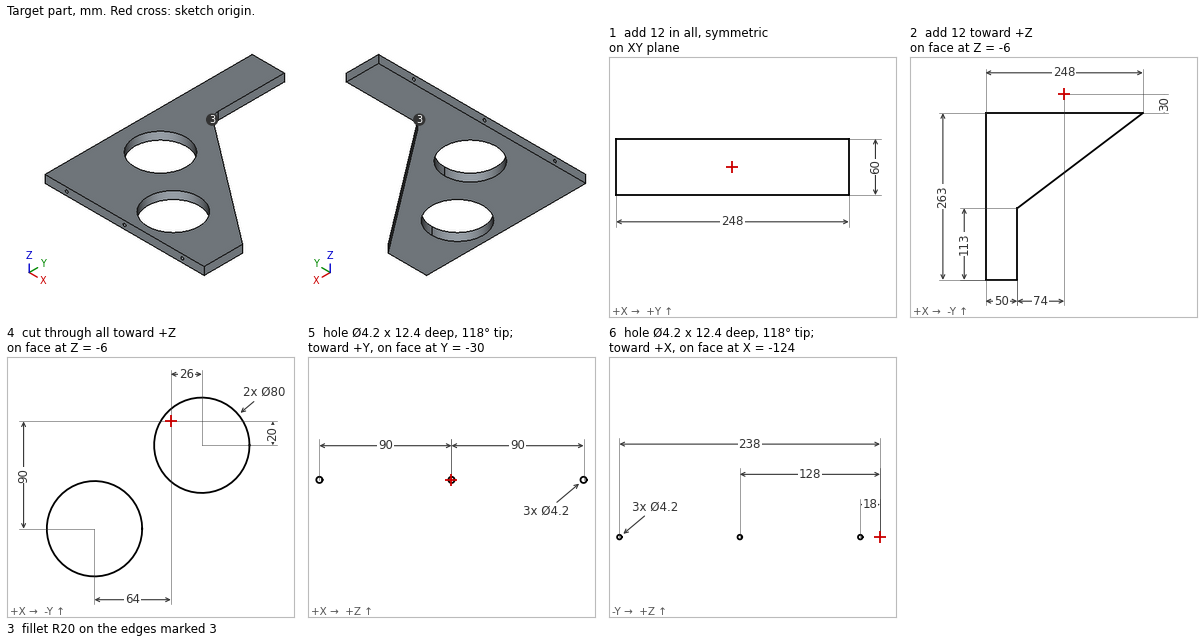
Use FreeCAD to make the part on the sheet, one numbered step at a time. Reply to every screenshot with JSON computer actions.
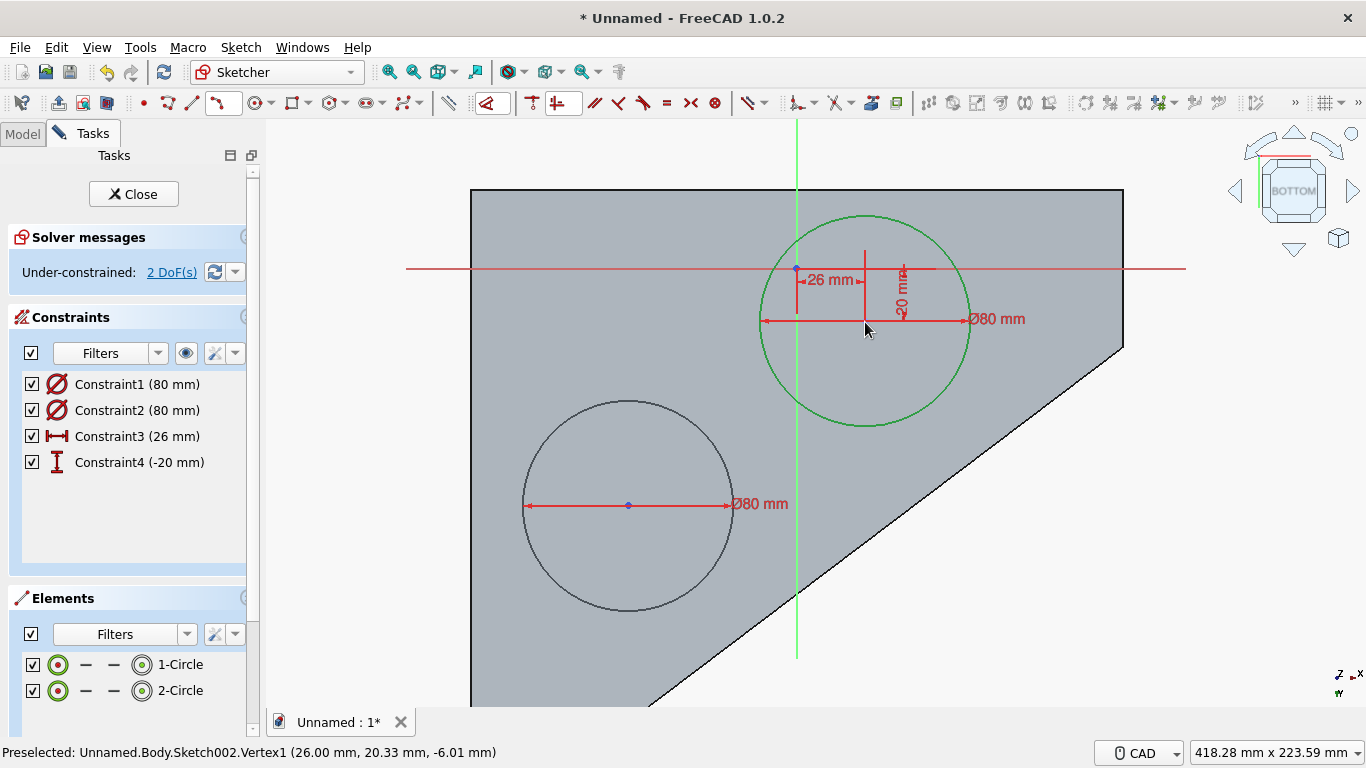
{"action": "left_click", "coordinate": [628, 506]}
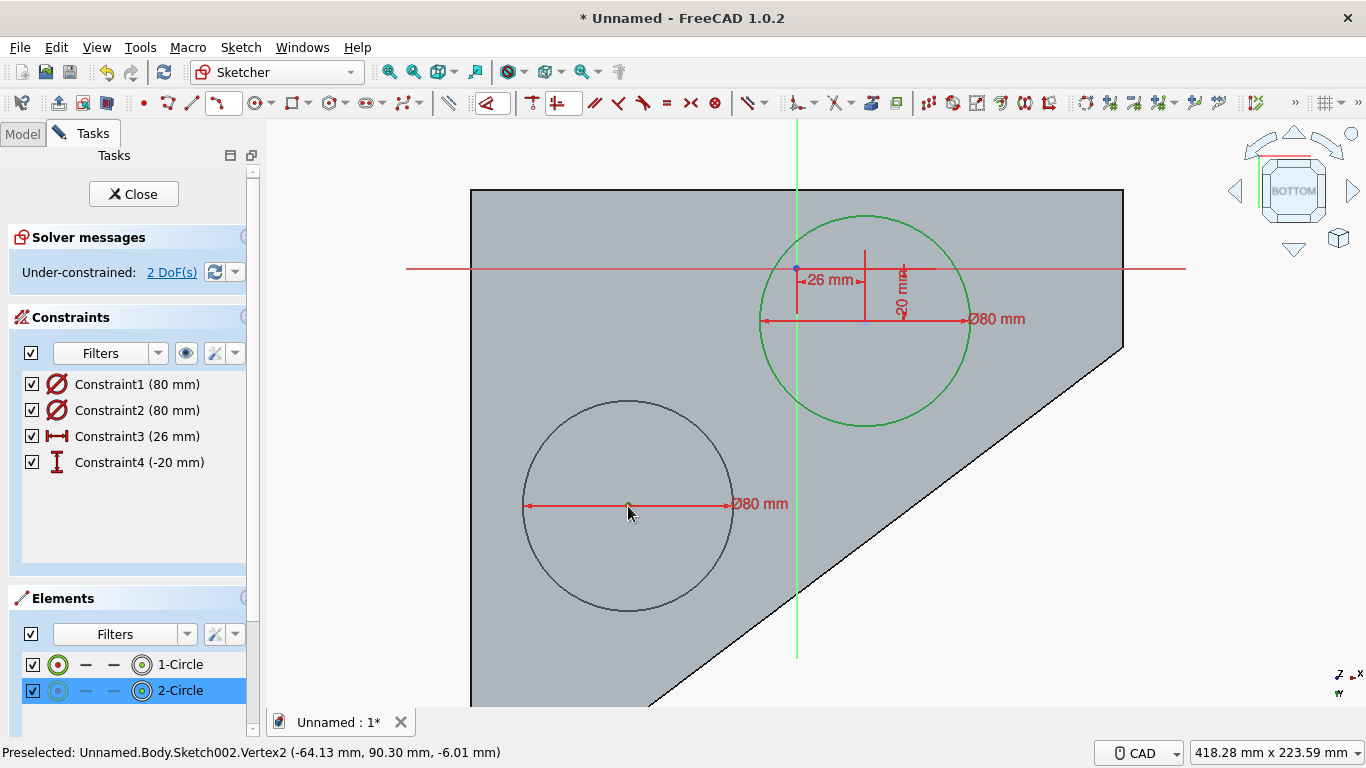
{"action": "key", "text": "l"}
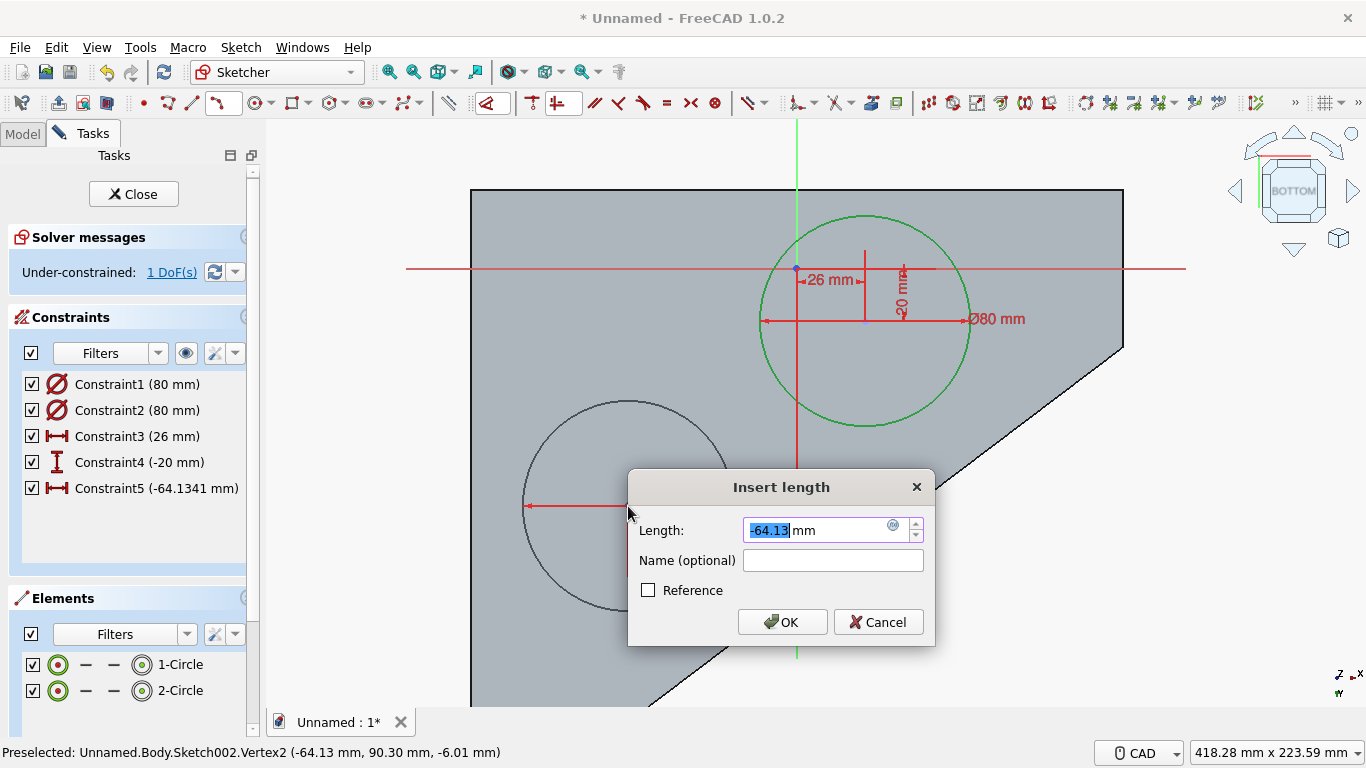
{"action": "type", "text": "-64"}
{"action": "key", "text": "Return"}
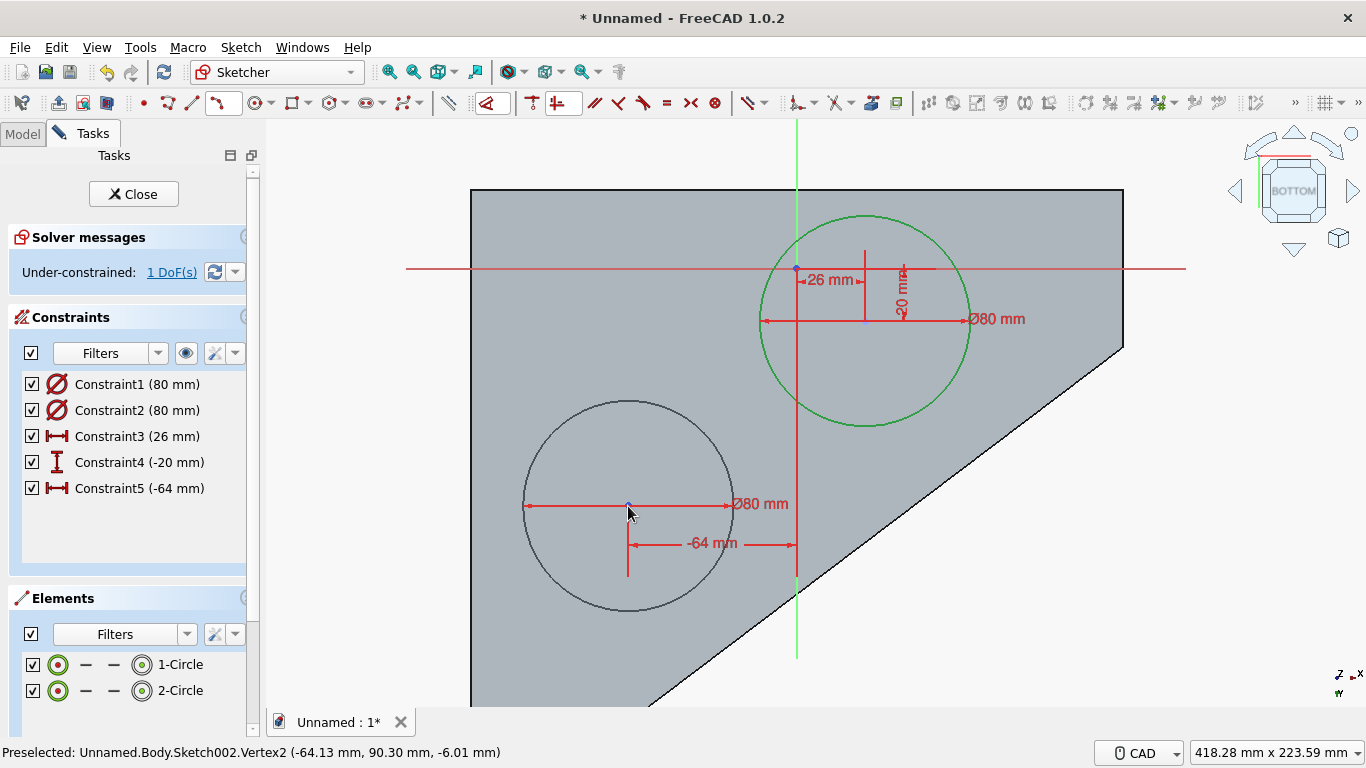
{"action": "left_click", "coordinate": [628, 506]}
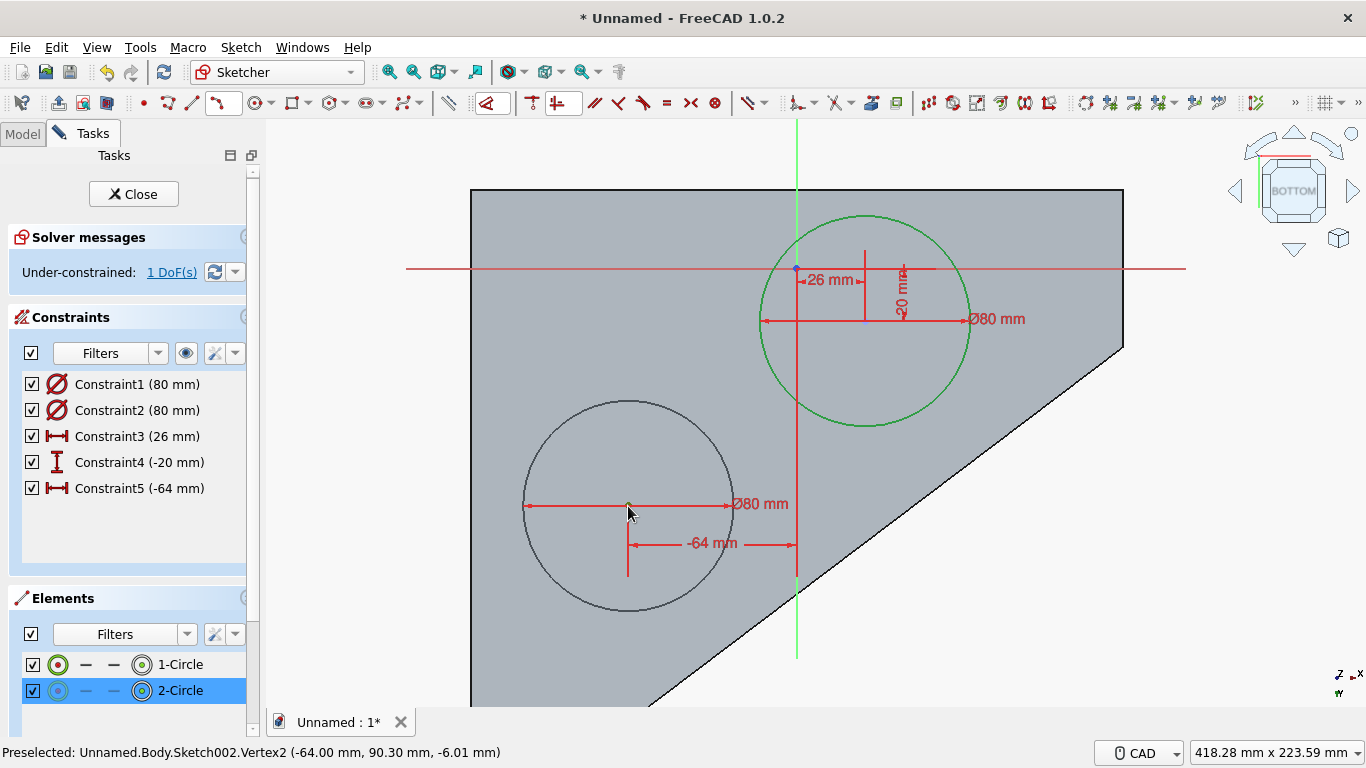
{"action": "key", "text": "i"}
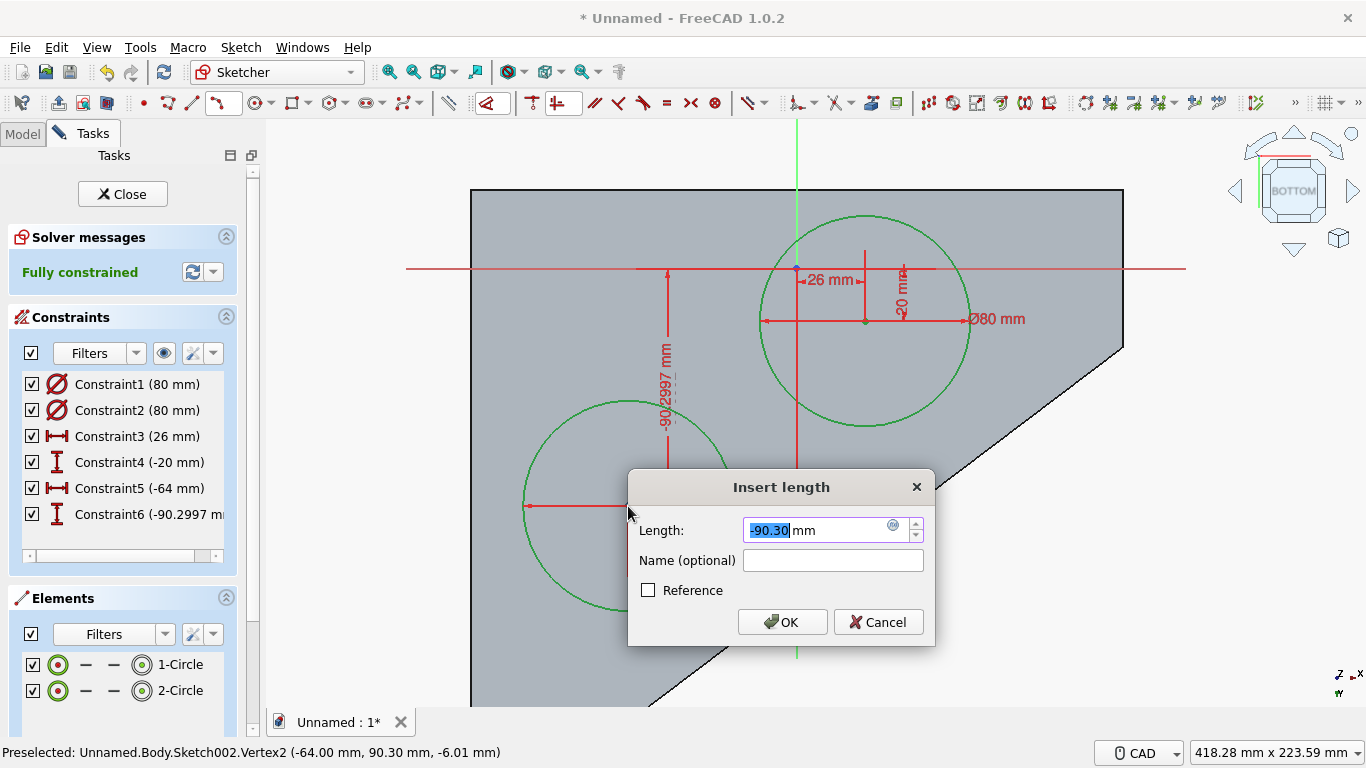
{"action": "type", "text": "-90"}
{"action": "key", "text": "Return"}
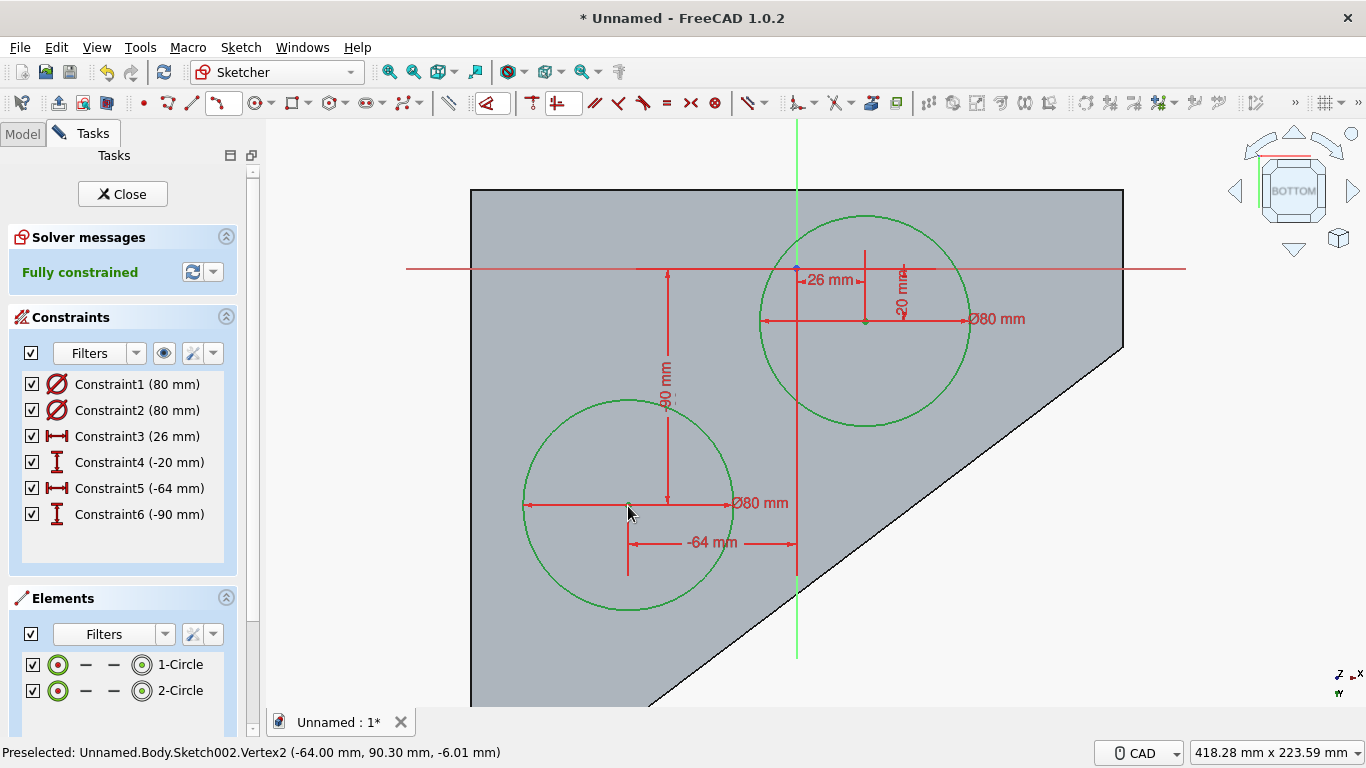
{"action": "left_click", "coordinate": [123, 194]}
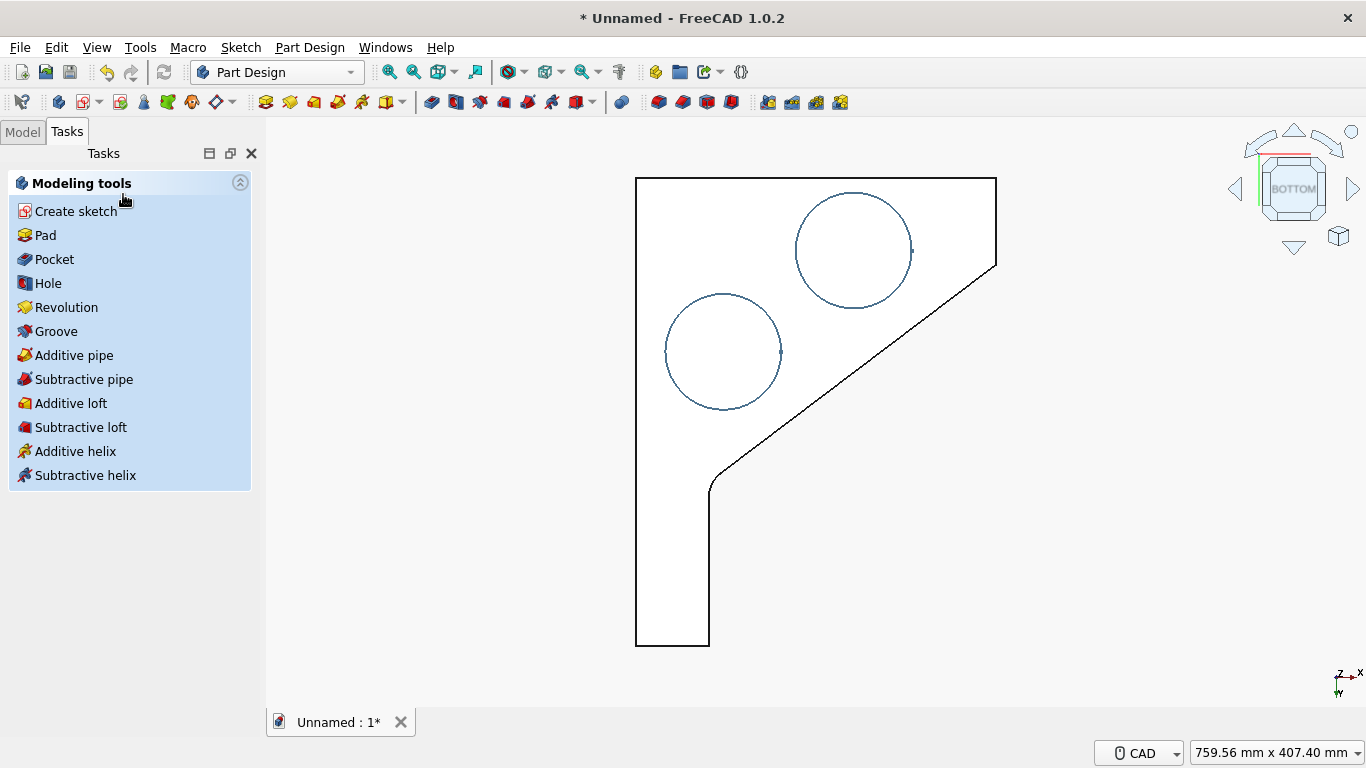
{"action": "left_click", "coordinate": [432, 102]}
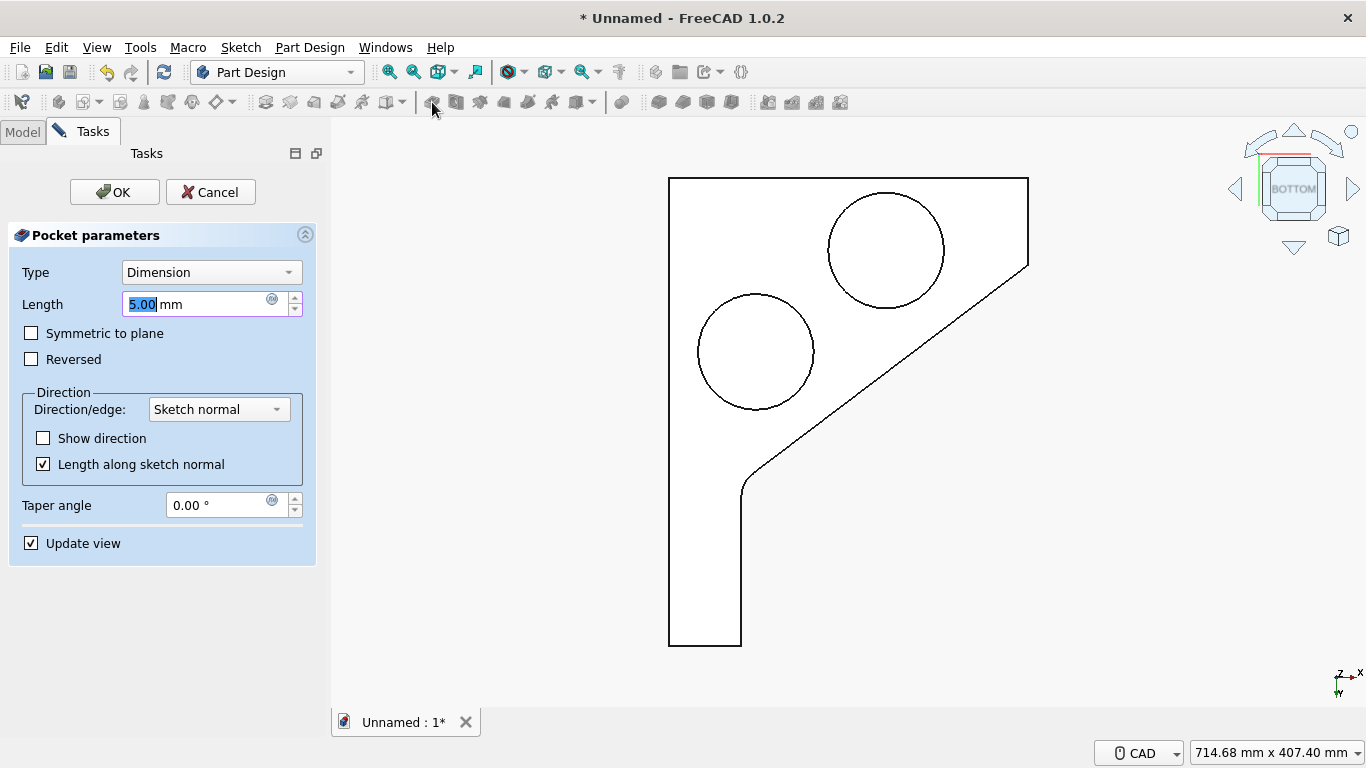
{"action": "left_click", "coordinate": [212, 272]}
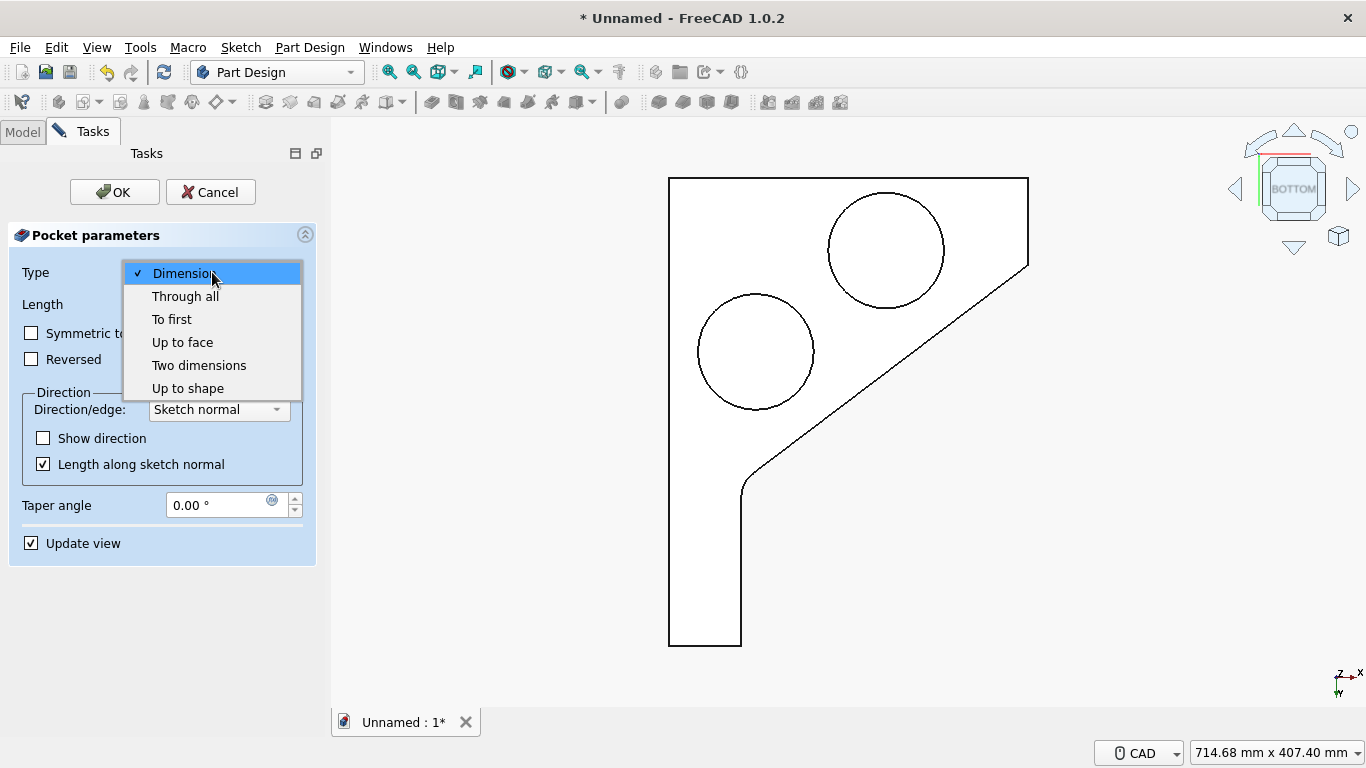
{"action": "left_click", "coordinate": [212, 296]}